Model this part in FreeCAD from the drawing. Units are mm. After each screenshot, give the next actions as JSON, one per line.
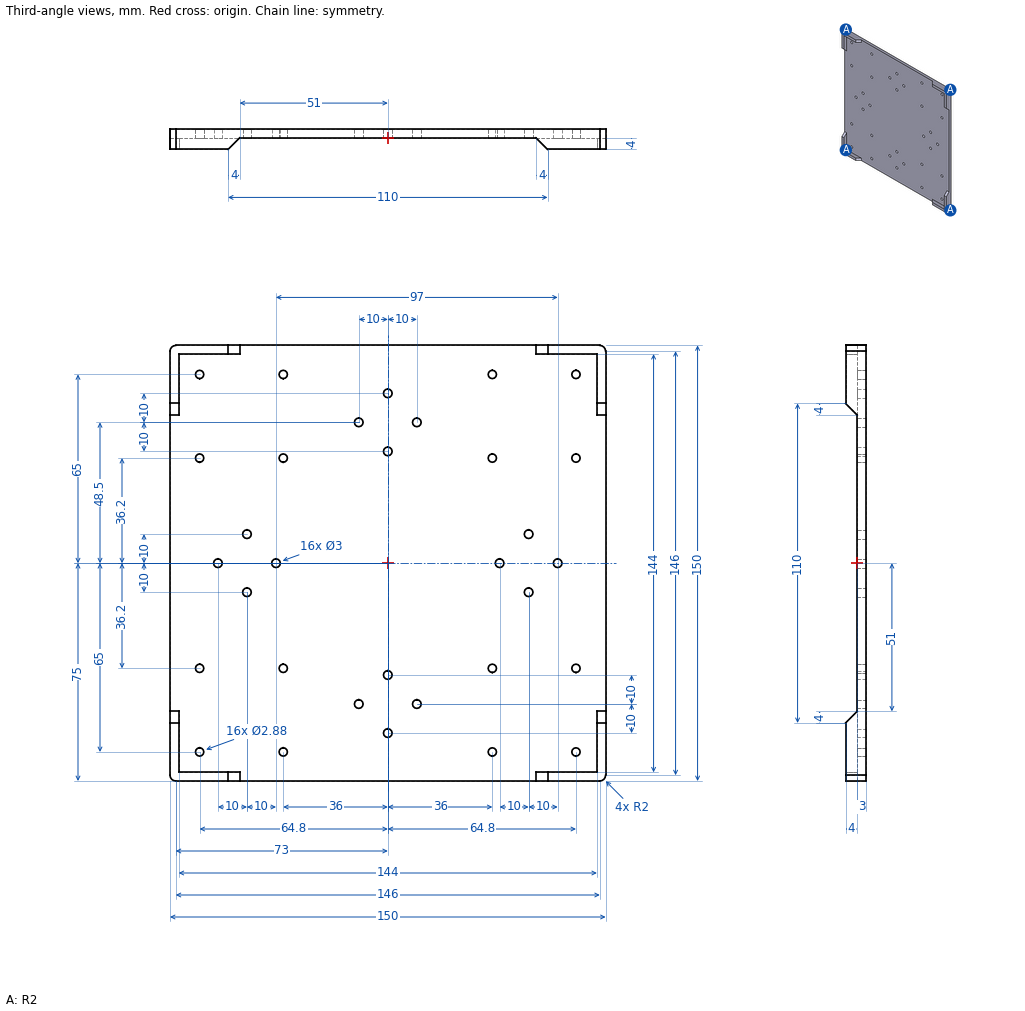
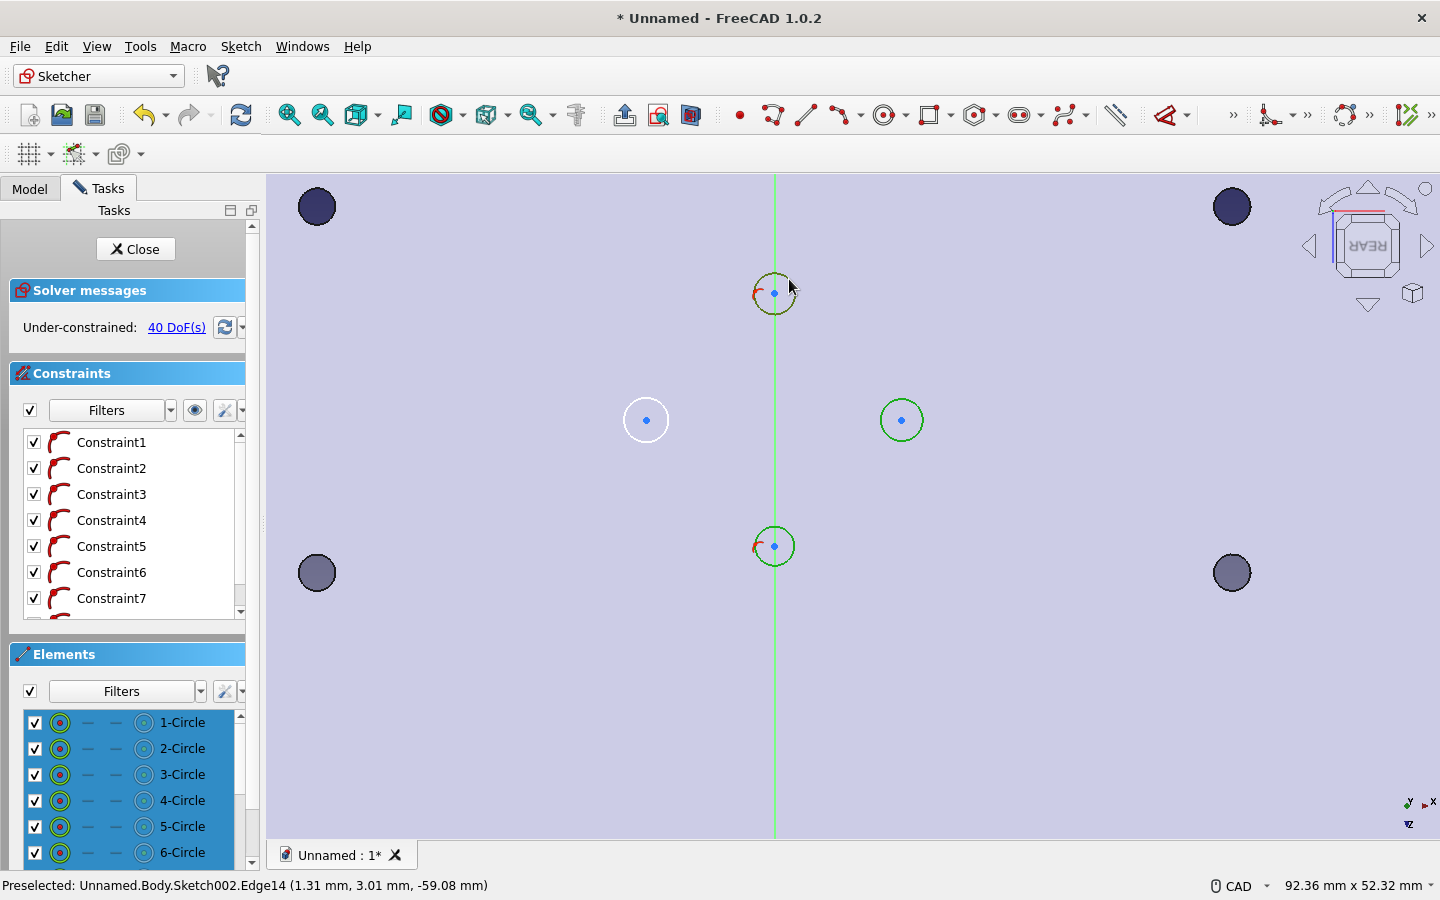
{"action": "left_click", "coordinate": [662, 404]}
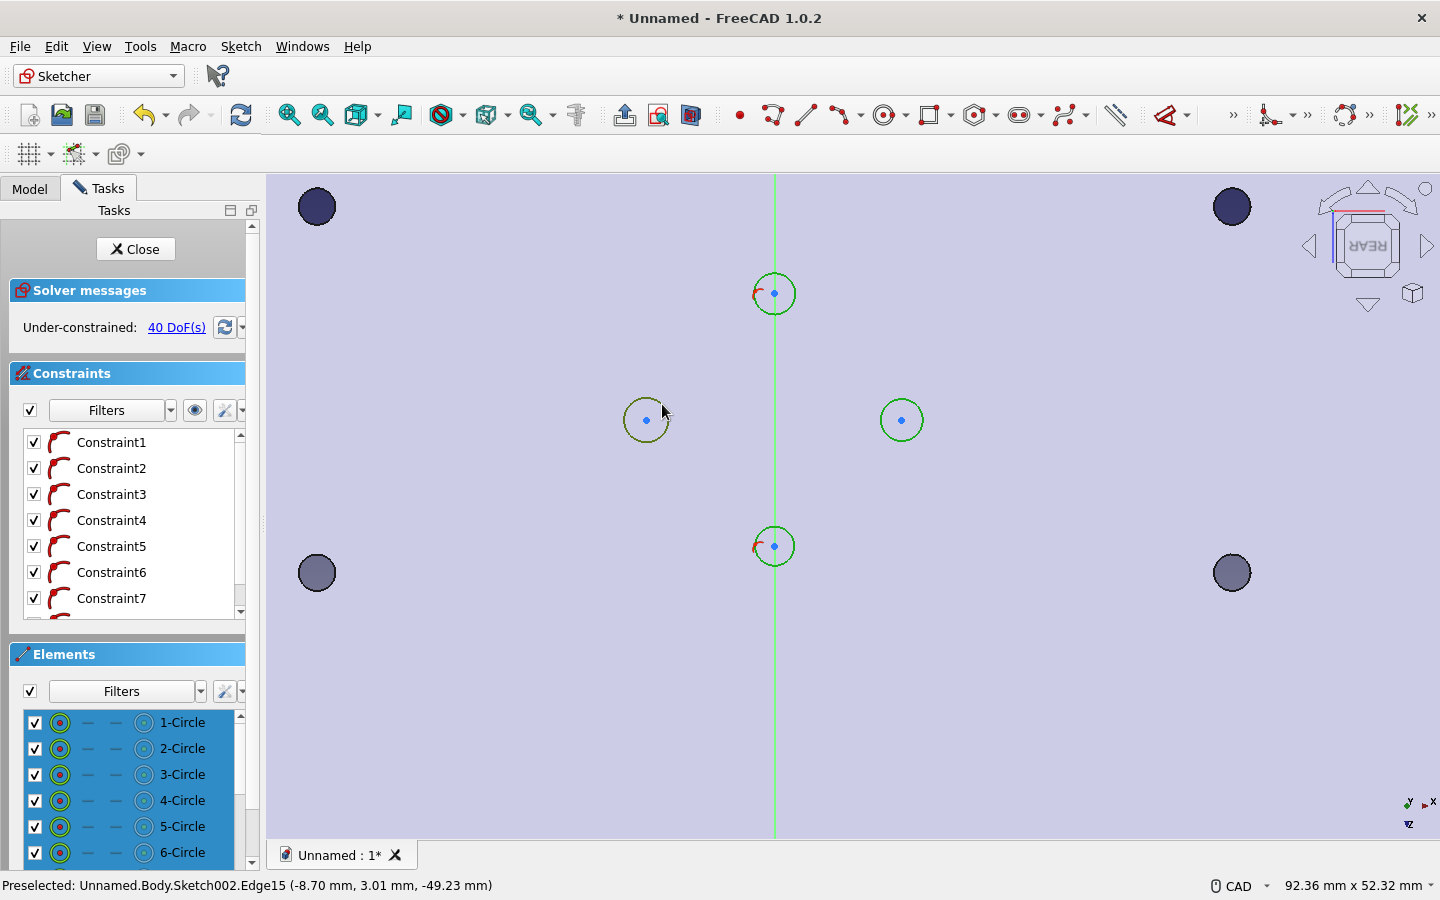
{"action": "scroll", "coordinate": [789, 280], "scroll_direction": "down", "scroll_amount": 6}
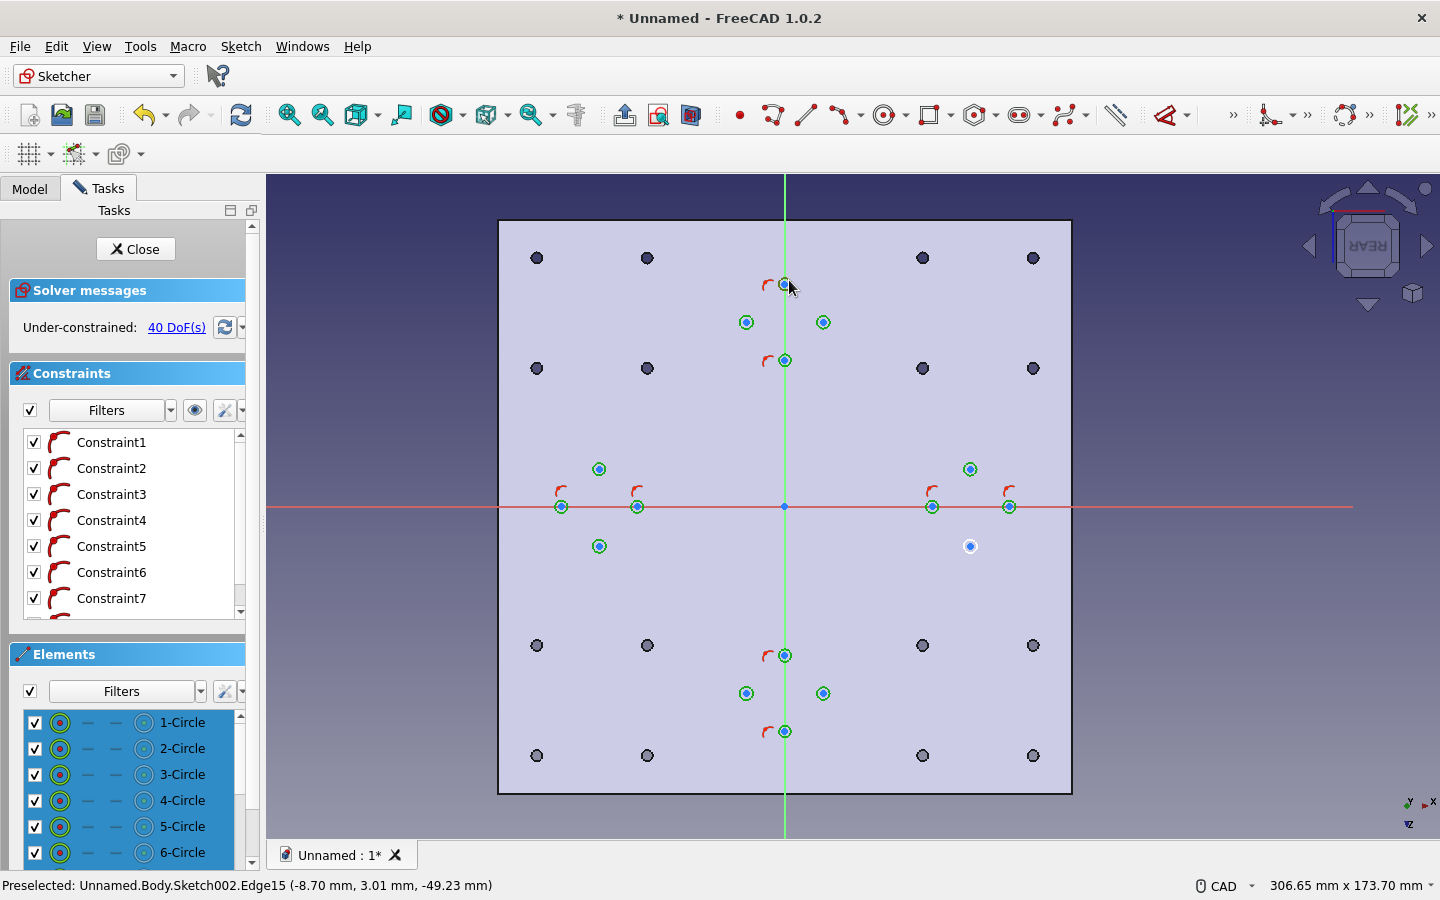
{"action": "scroll", "coordinate": [975, 542], "scroll_direction": "up", "scroll_amount": 4}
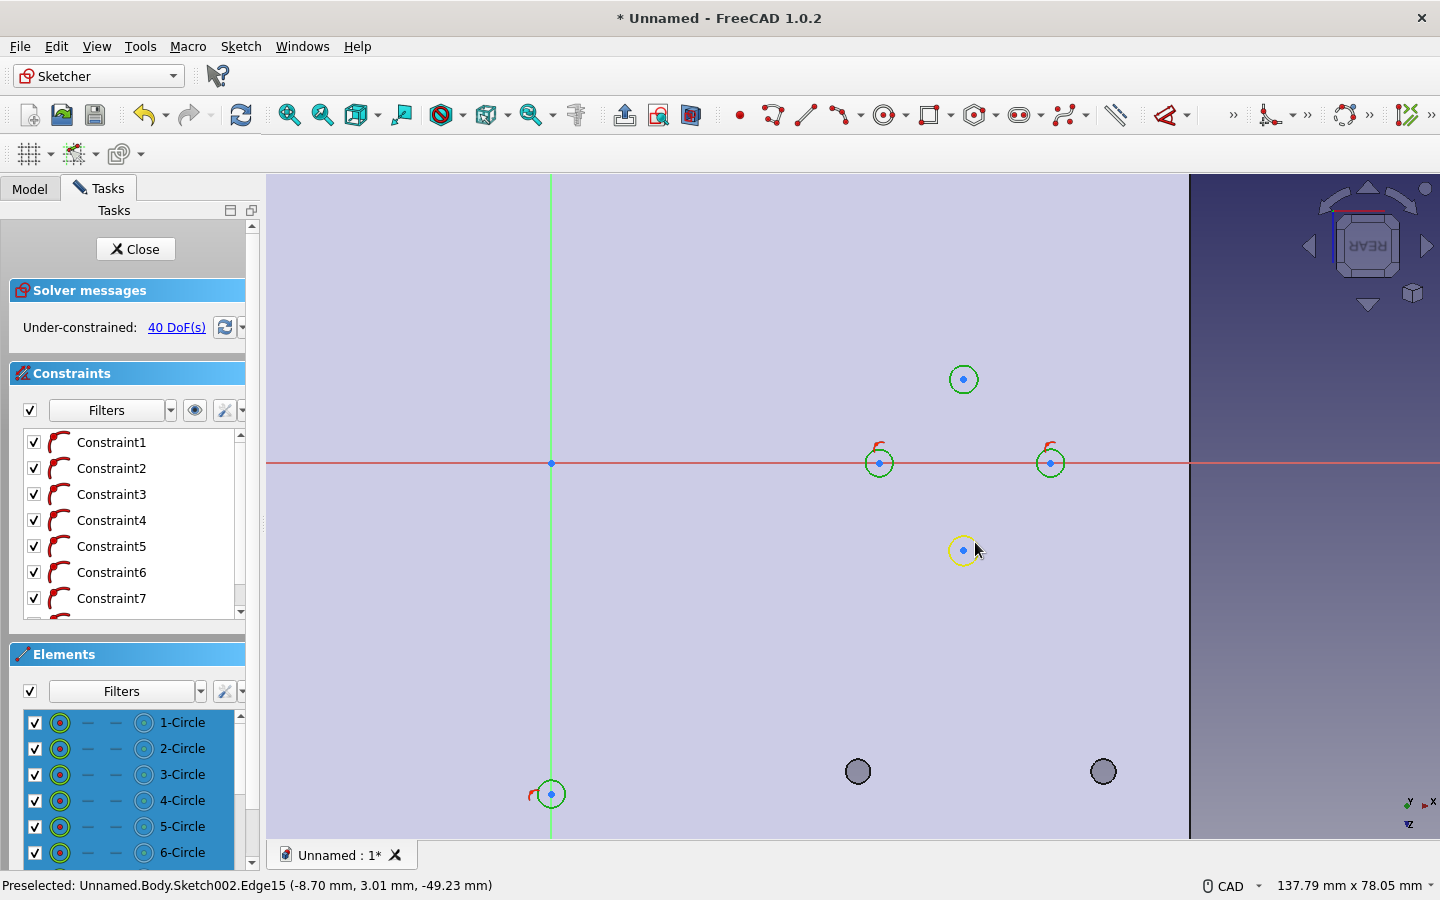
{"action": "left_click", "coordinate": [974, 540]}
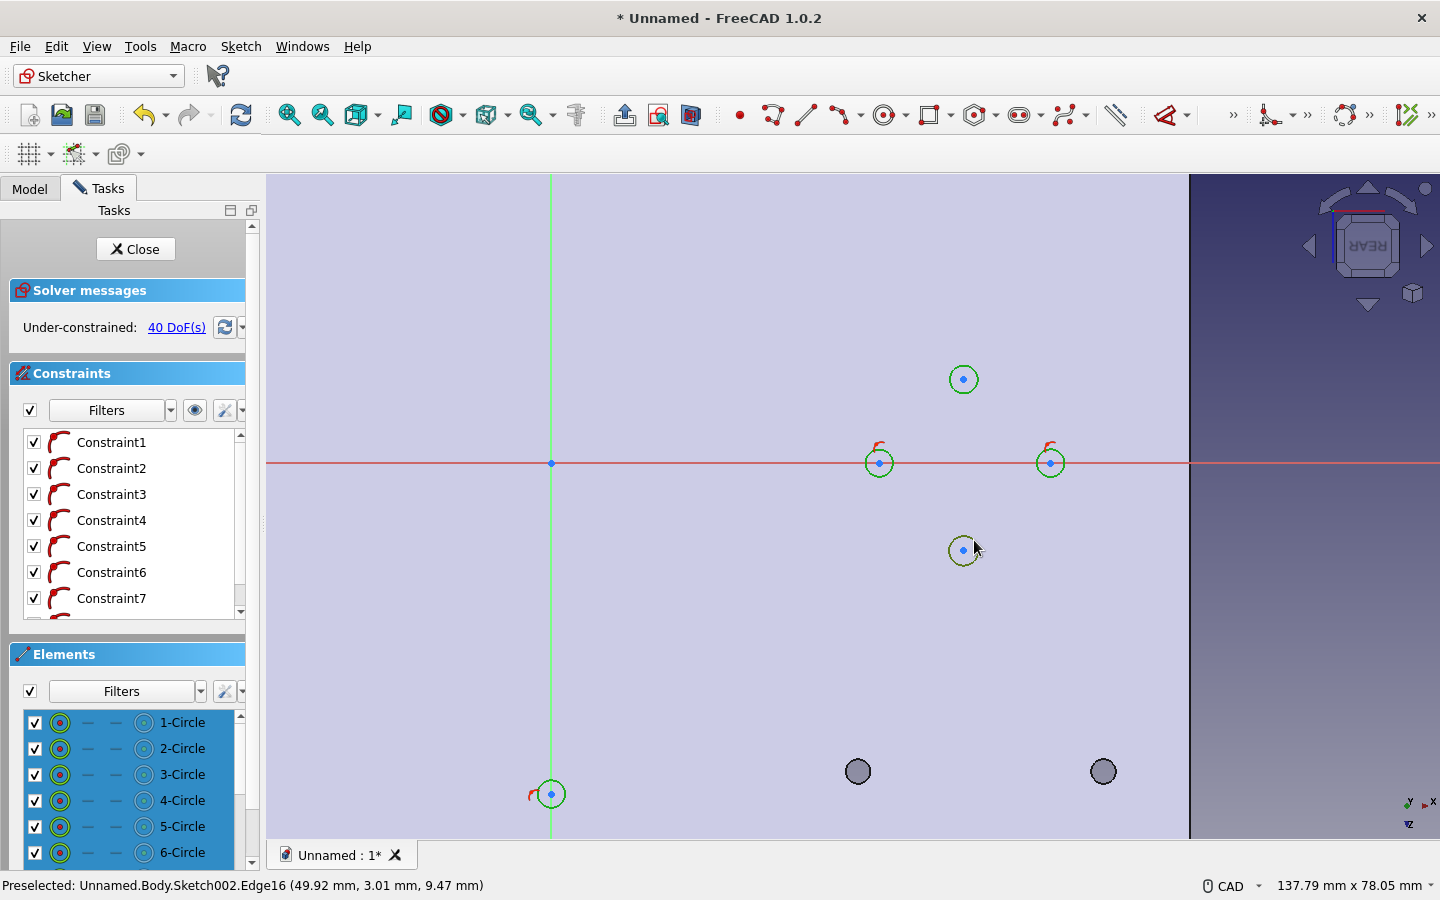
{"action": "key", "text": "e"}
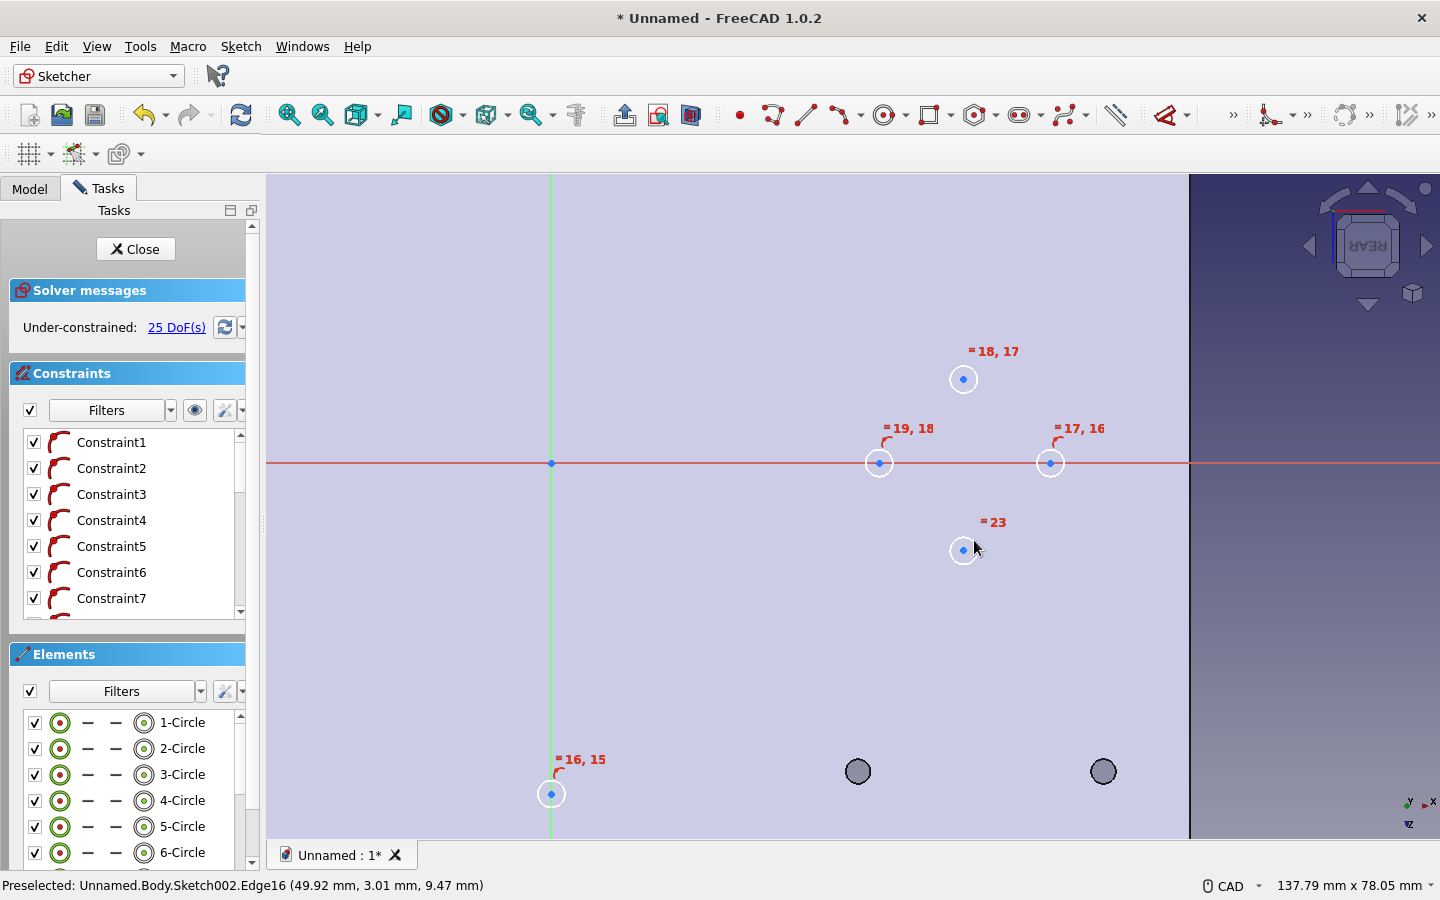
{"action": "scroll", "coordinate": [975, 542], "scroll_direction": "down", "scroll_amount": 4}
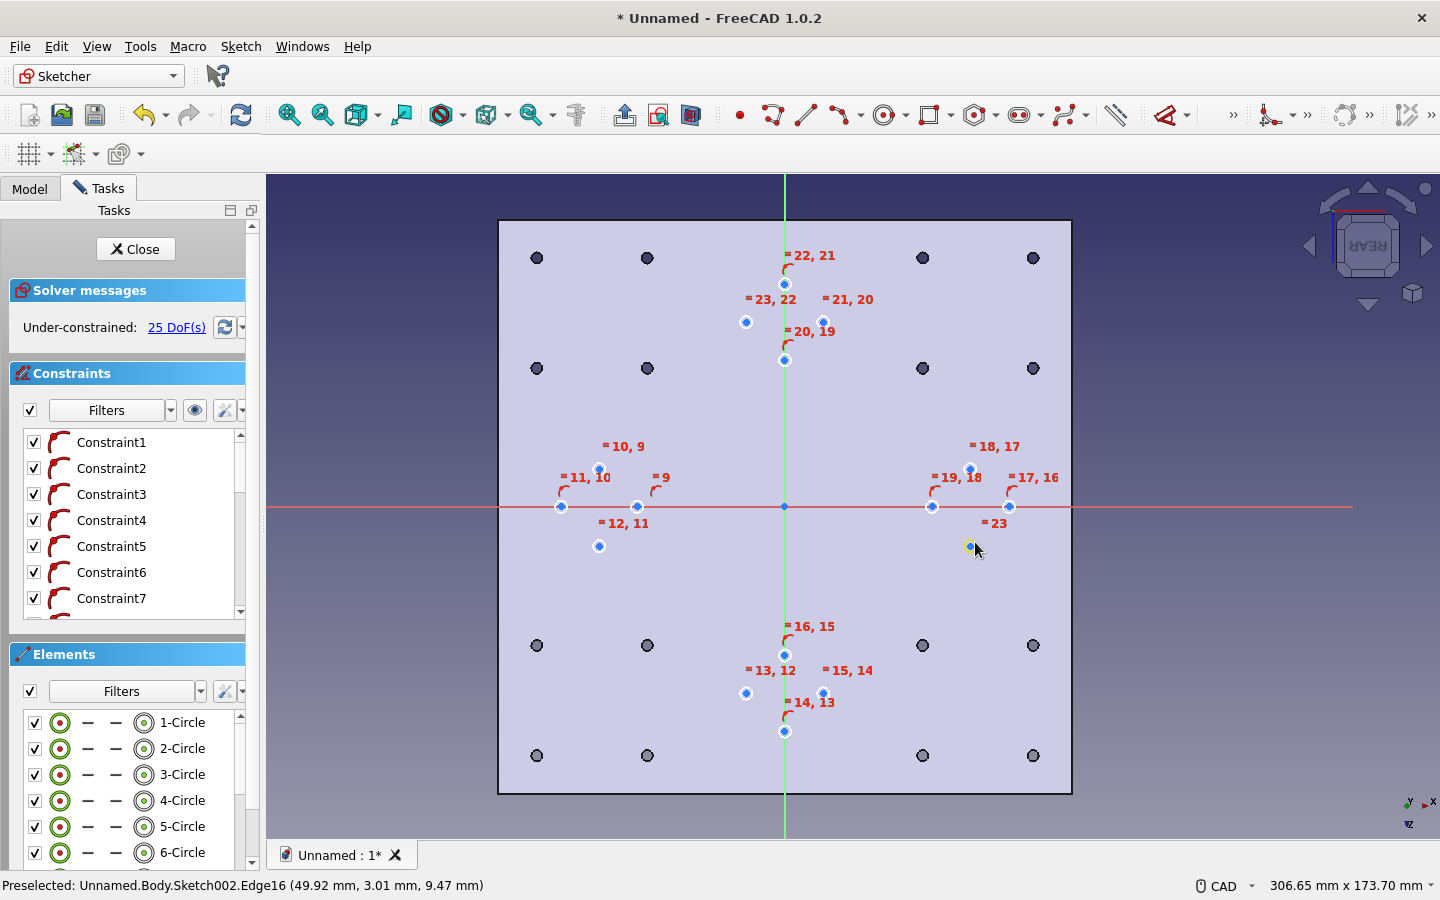
{"action": "left_click", "coordinate": [599, 469]}